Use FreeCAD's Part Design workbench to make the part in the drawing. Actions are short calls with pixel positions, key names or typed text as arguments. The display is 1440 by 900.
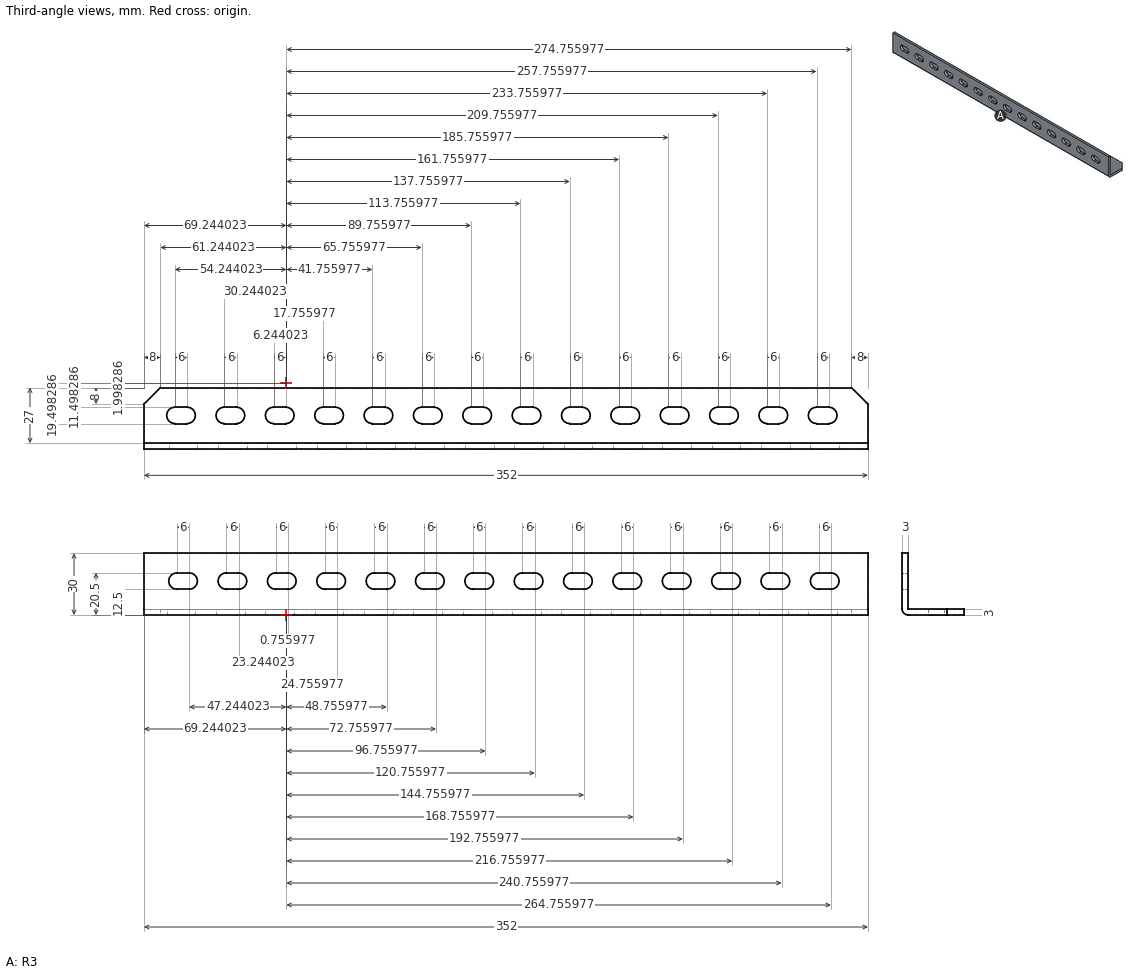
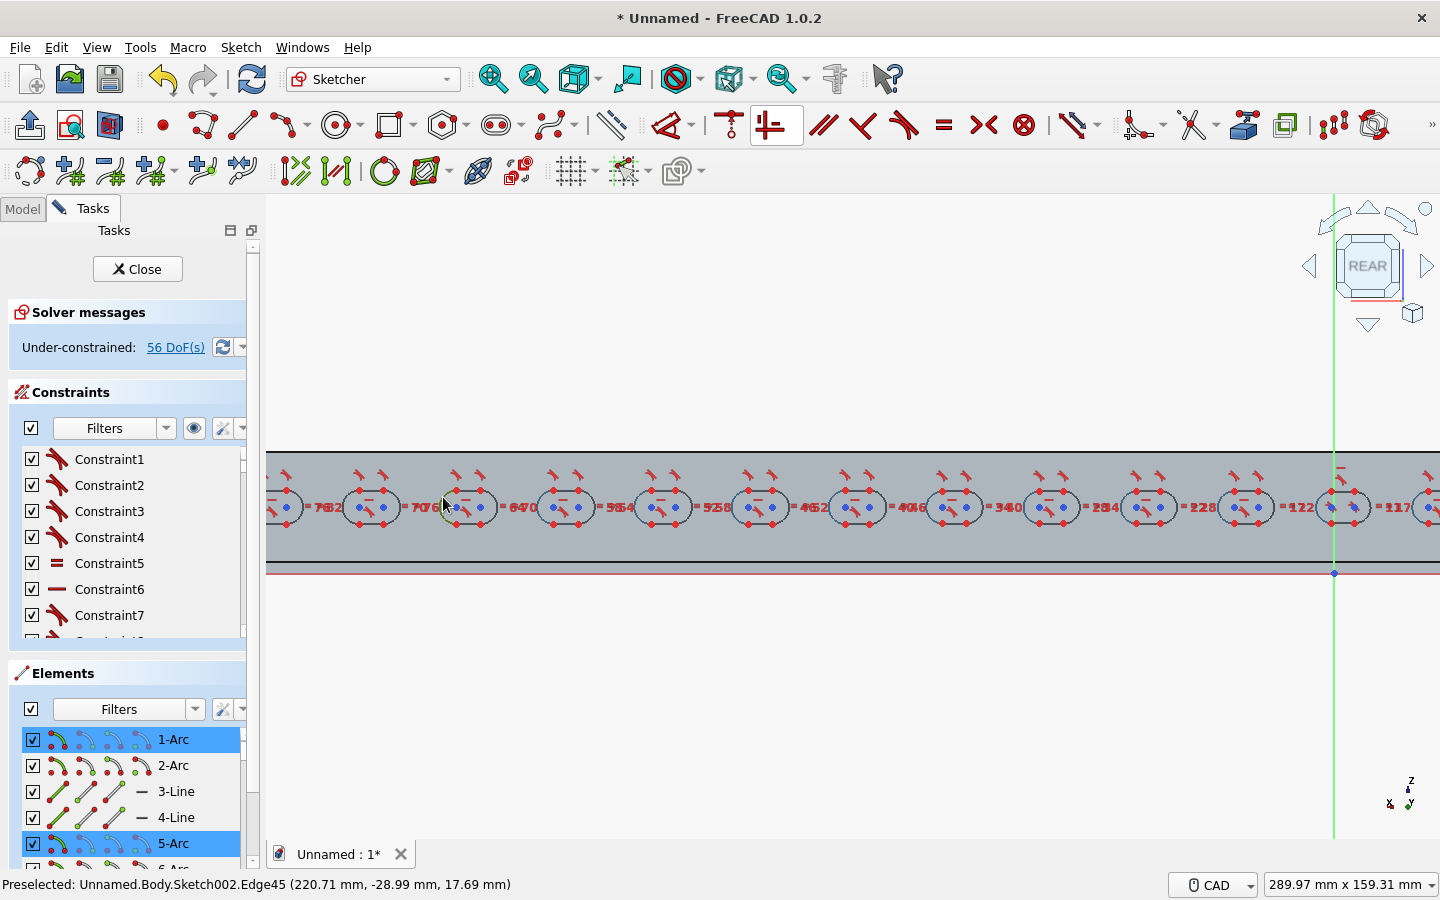
click(346, 497)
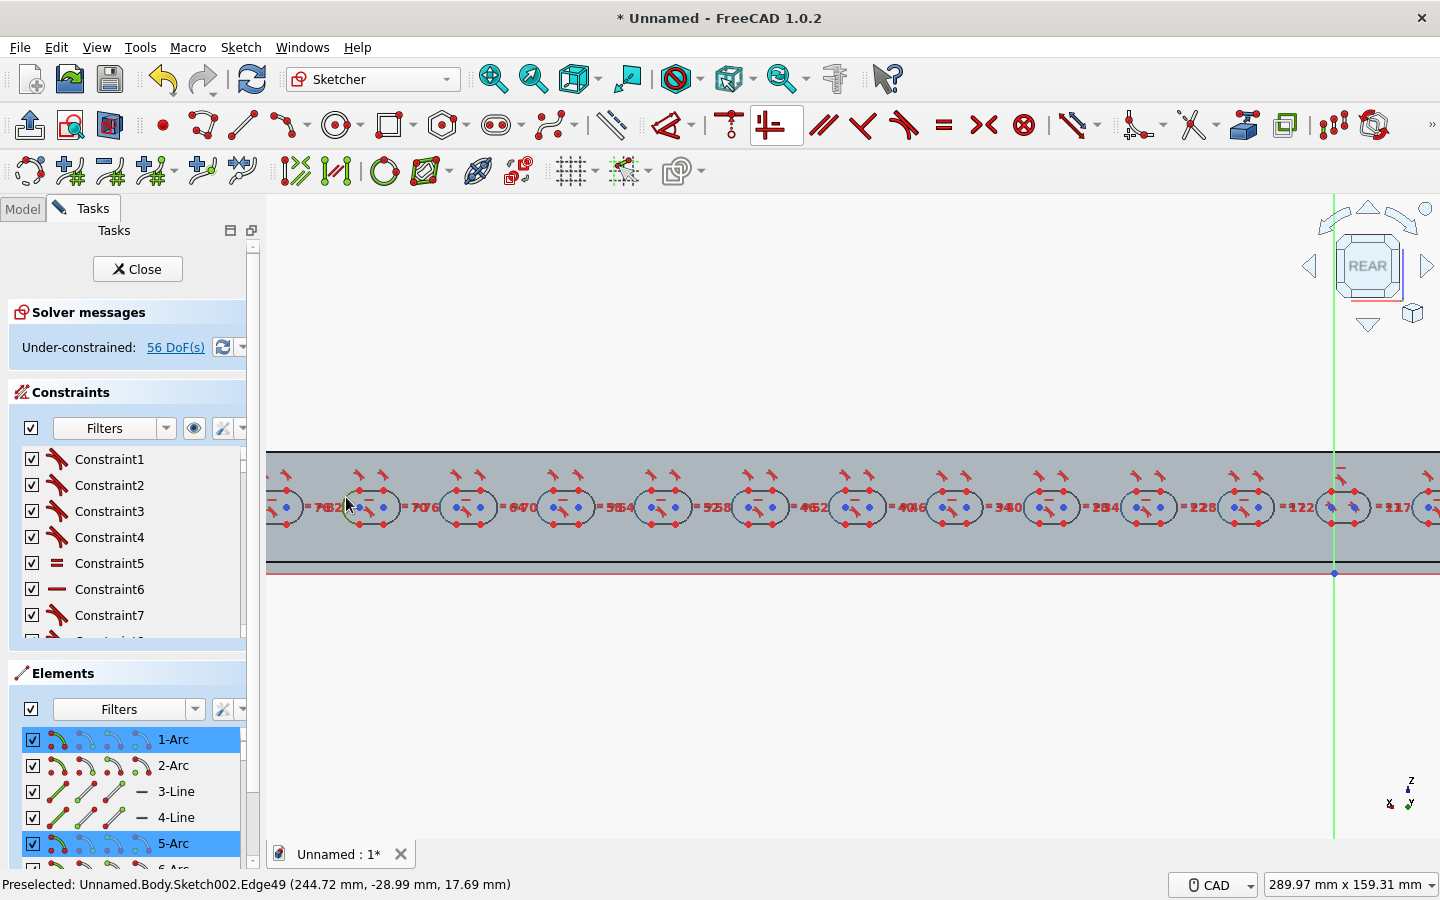
scroll(637, 497, down, 3)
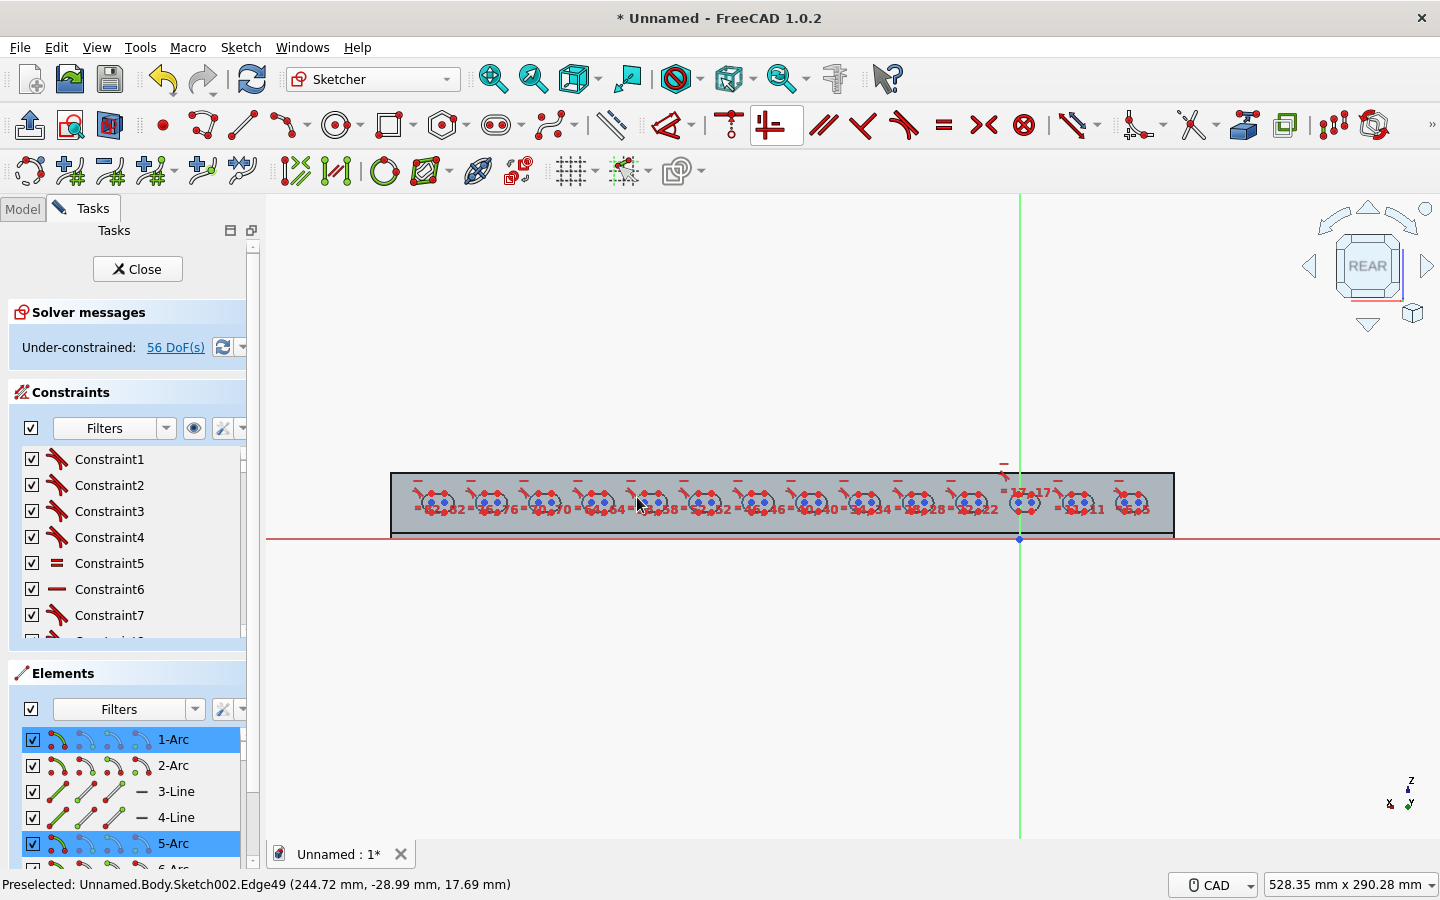
scroll(424, 497, up, 3)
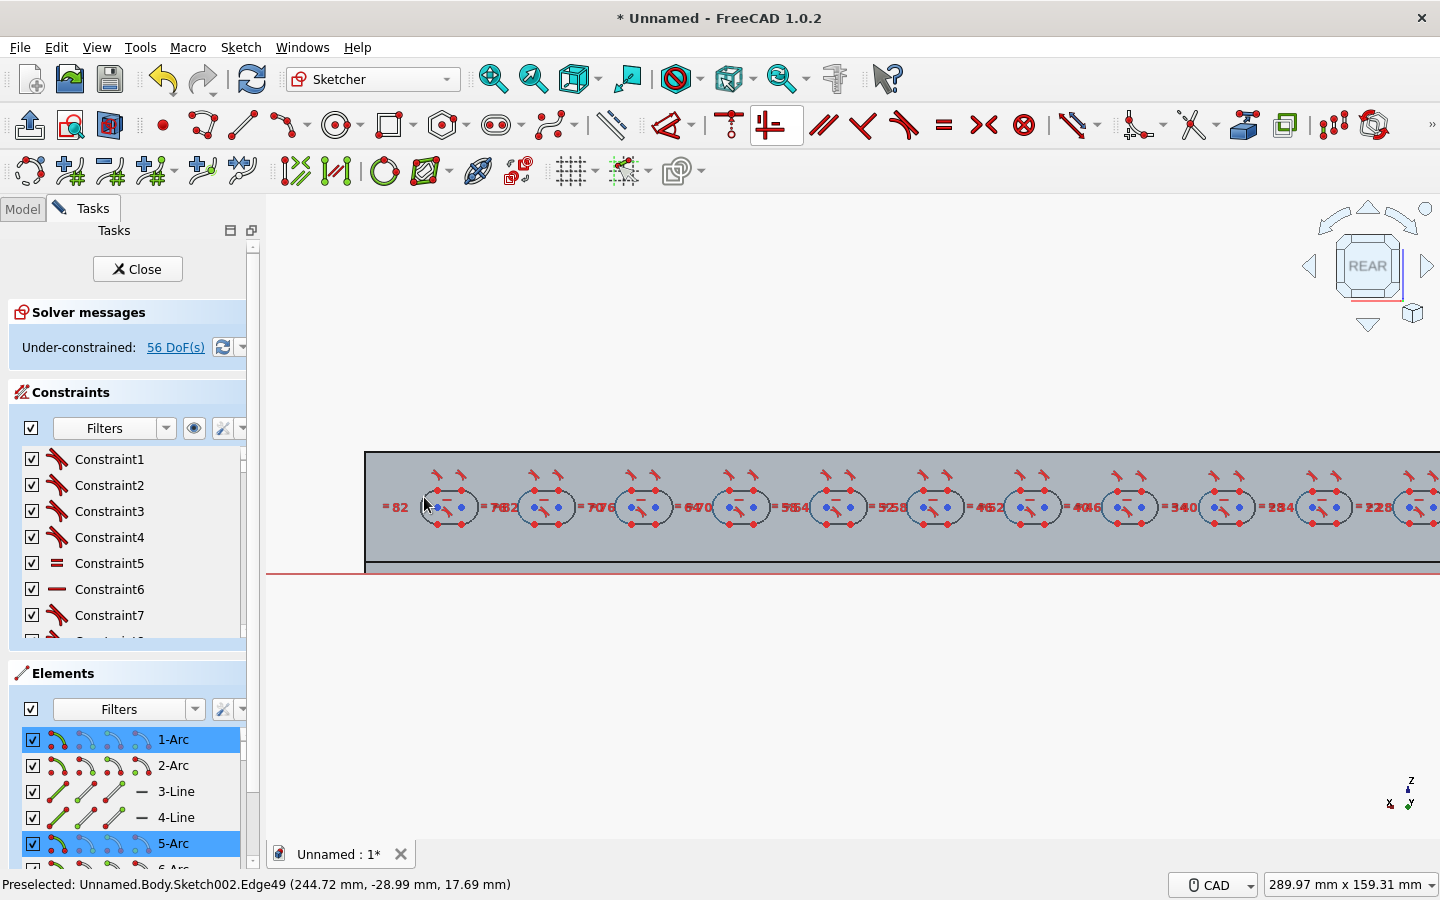
click(424, 497)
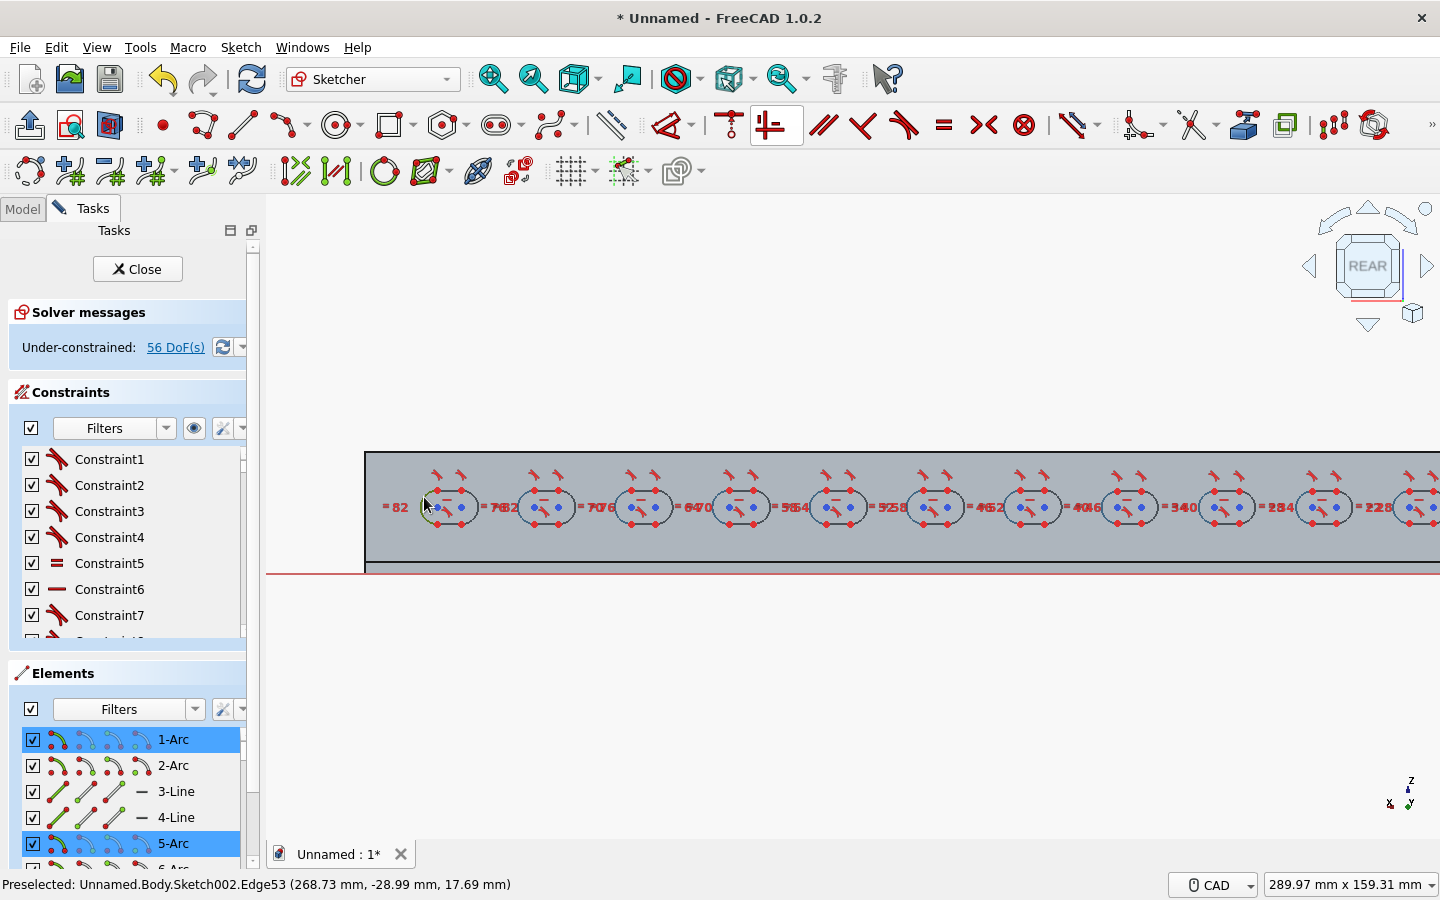
click(944, 126)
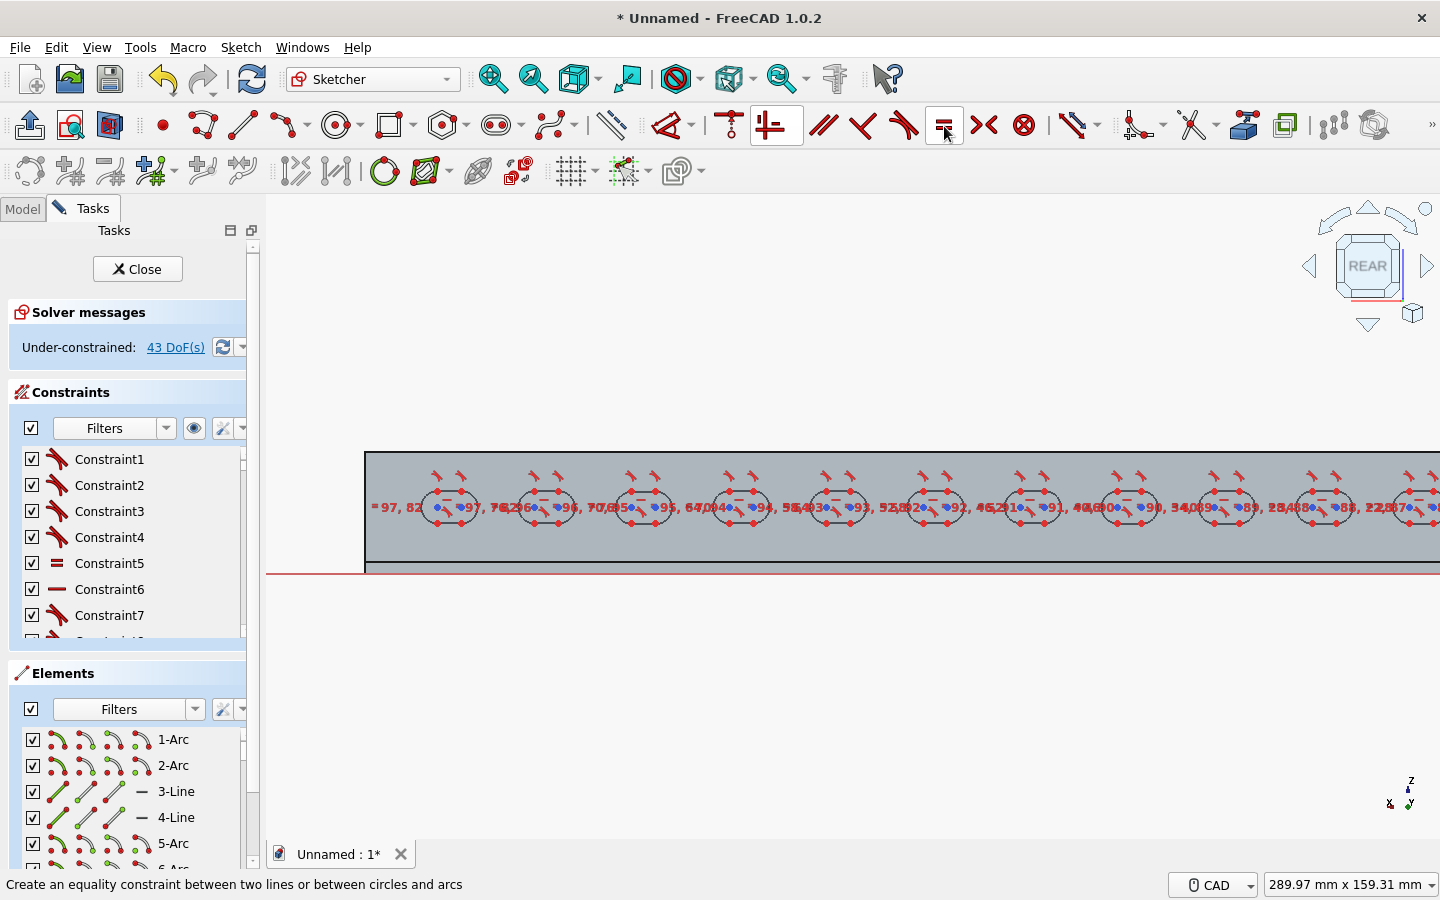
click(666, 126)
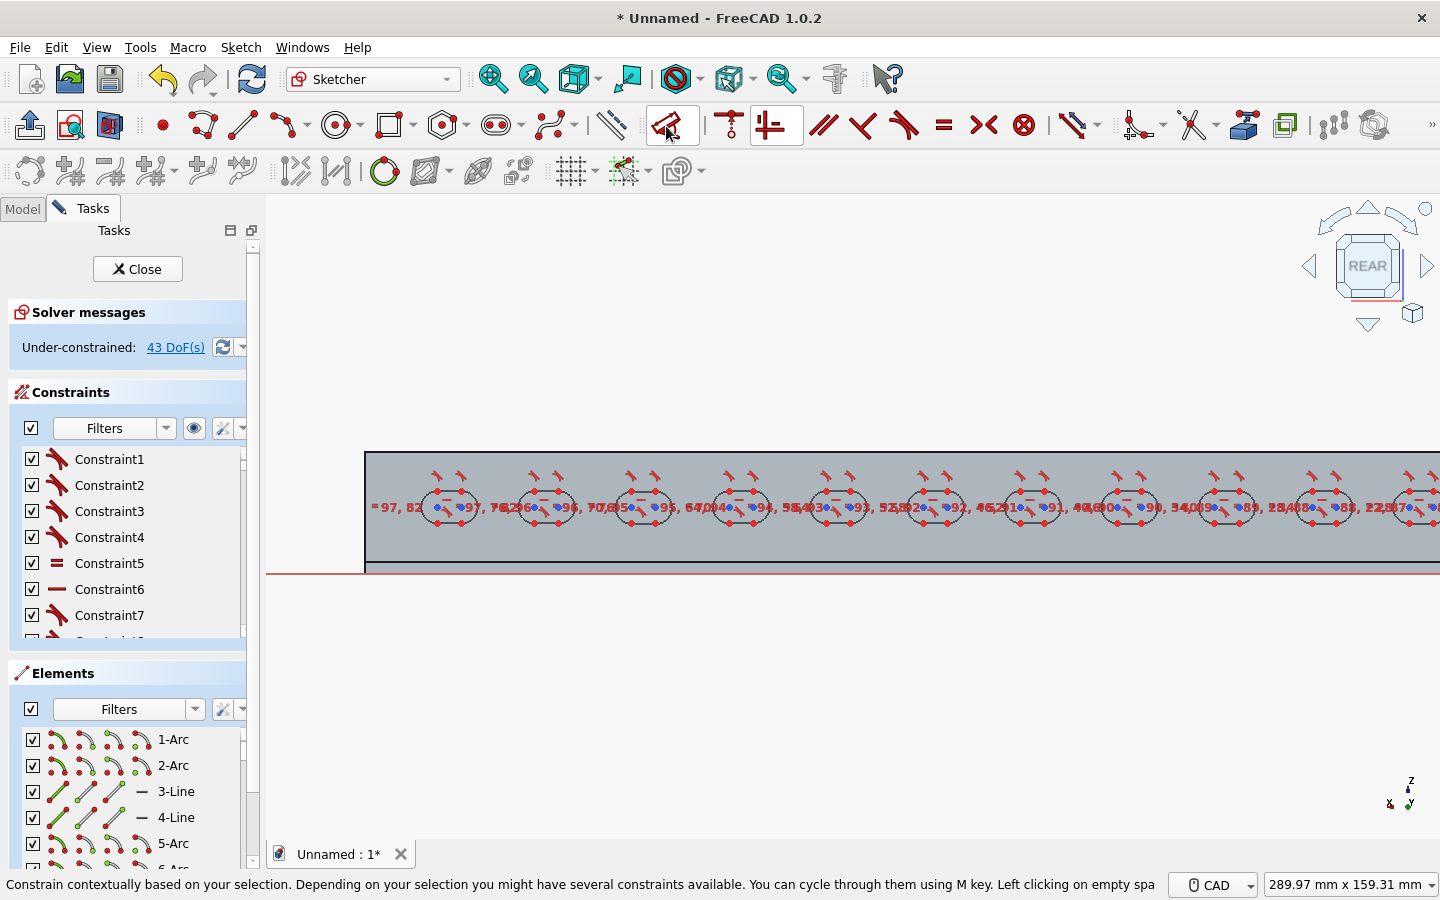
scroll(424, 497, down, 3)